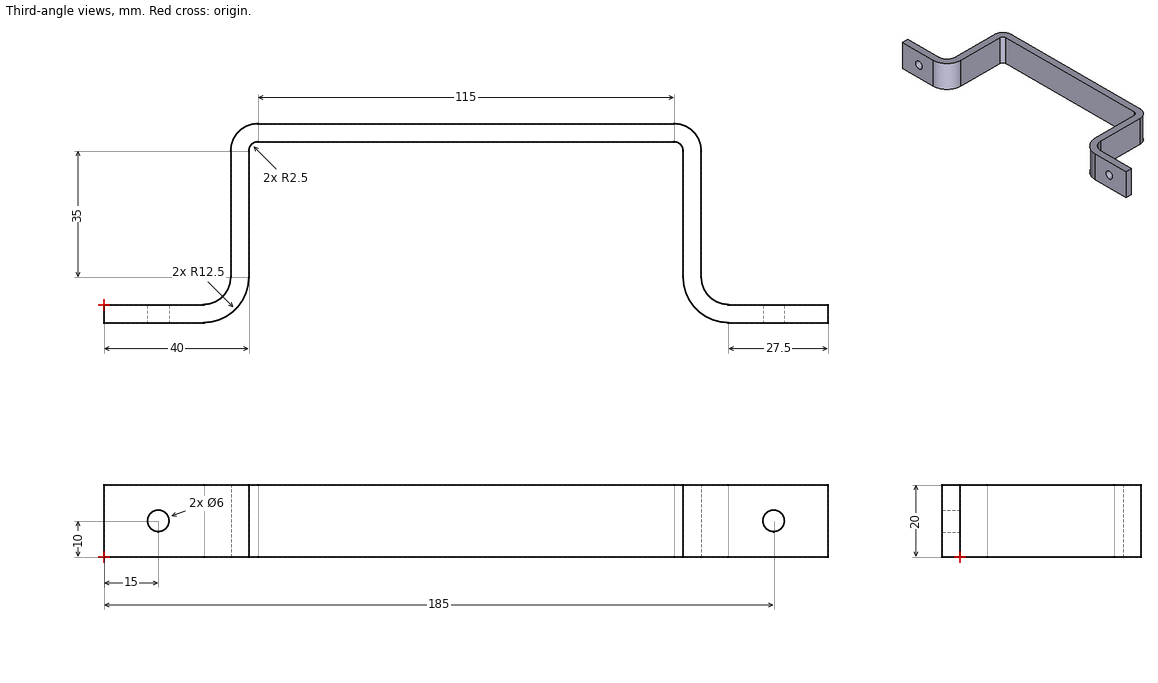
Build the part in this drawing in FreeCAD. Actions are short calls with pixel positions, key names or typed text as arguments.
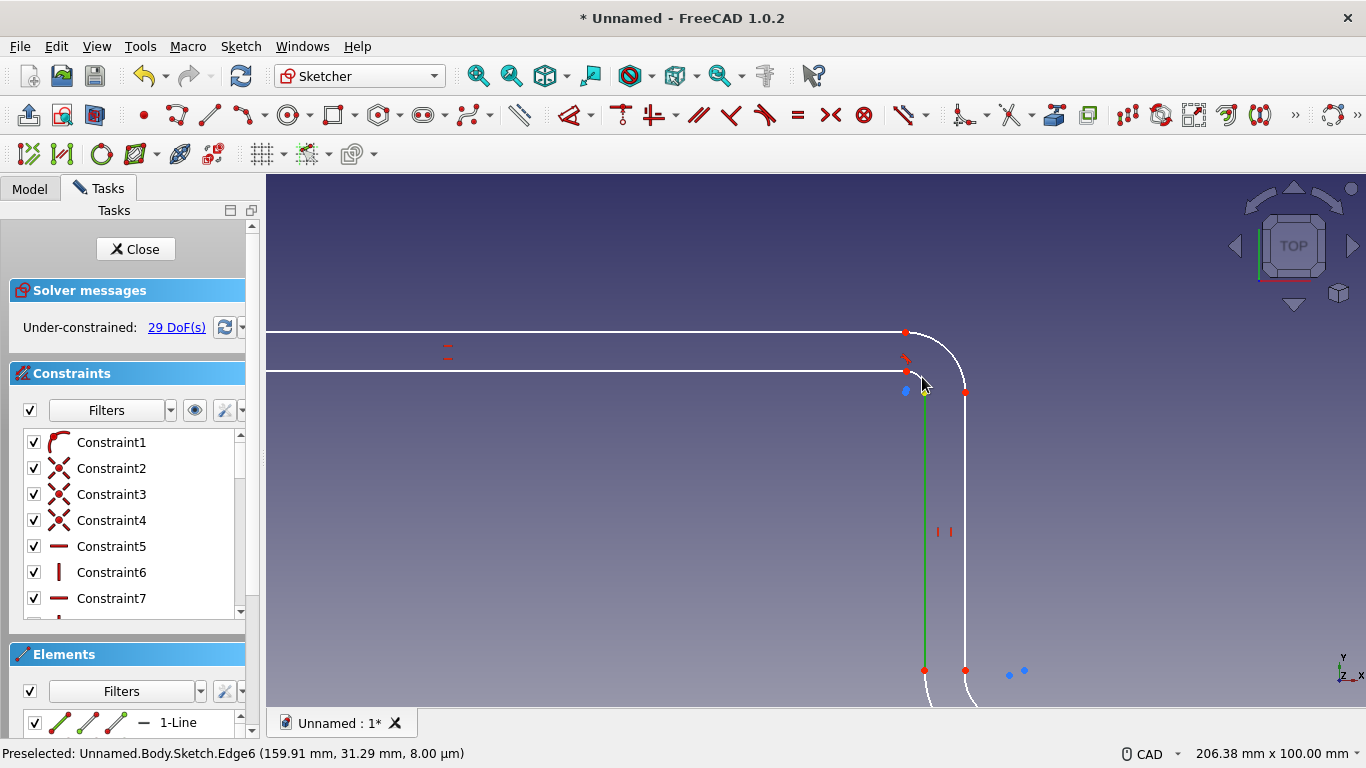
click(920, 378)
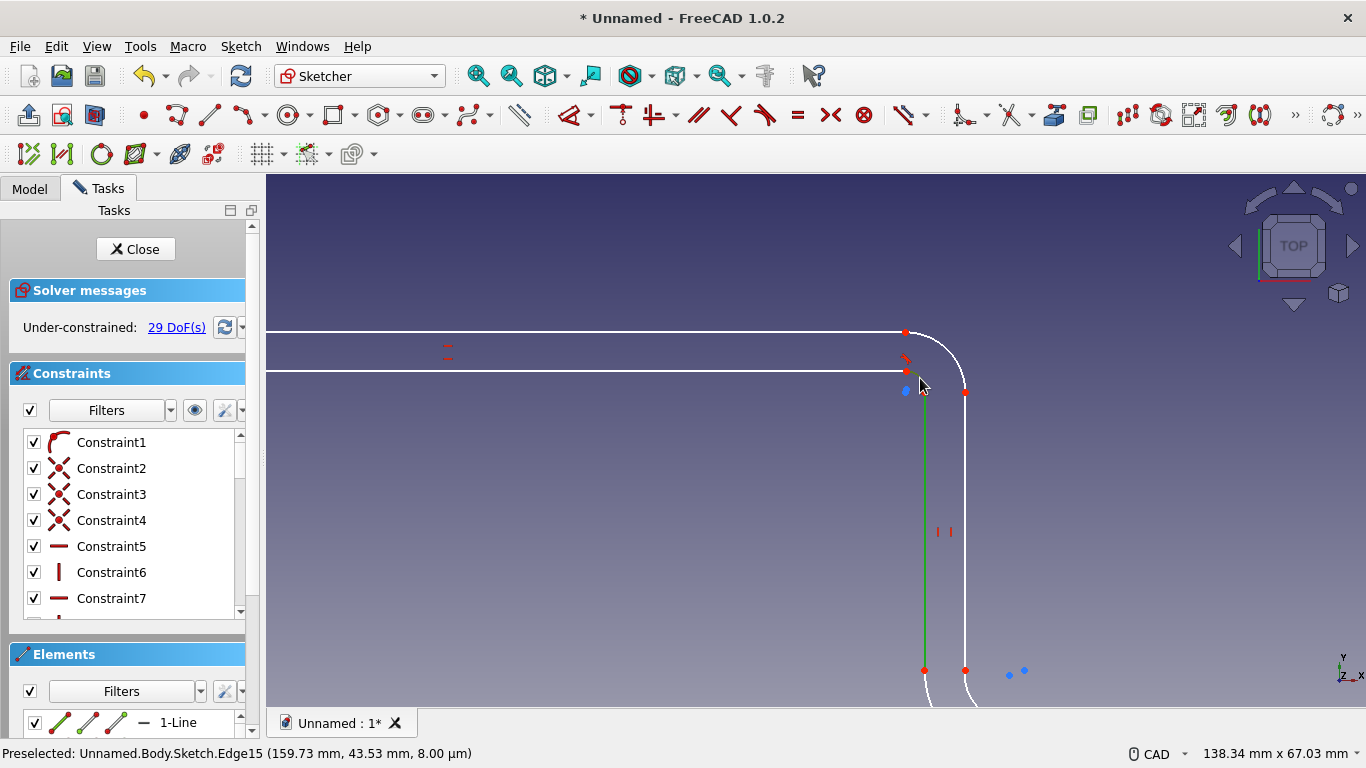
click(765, 116)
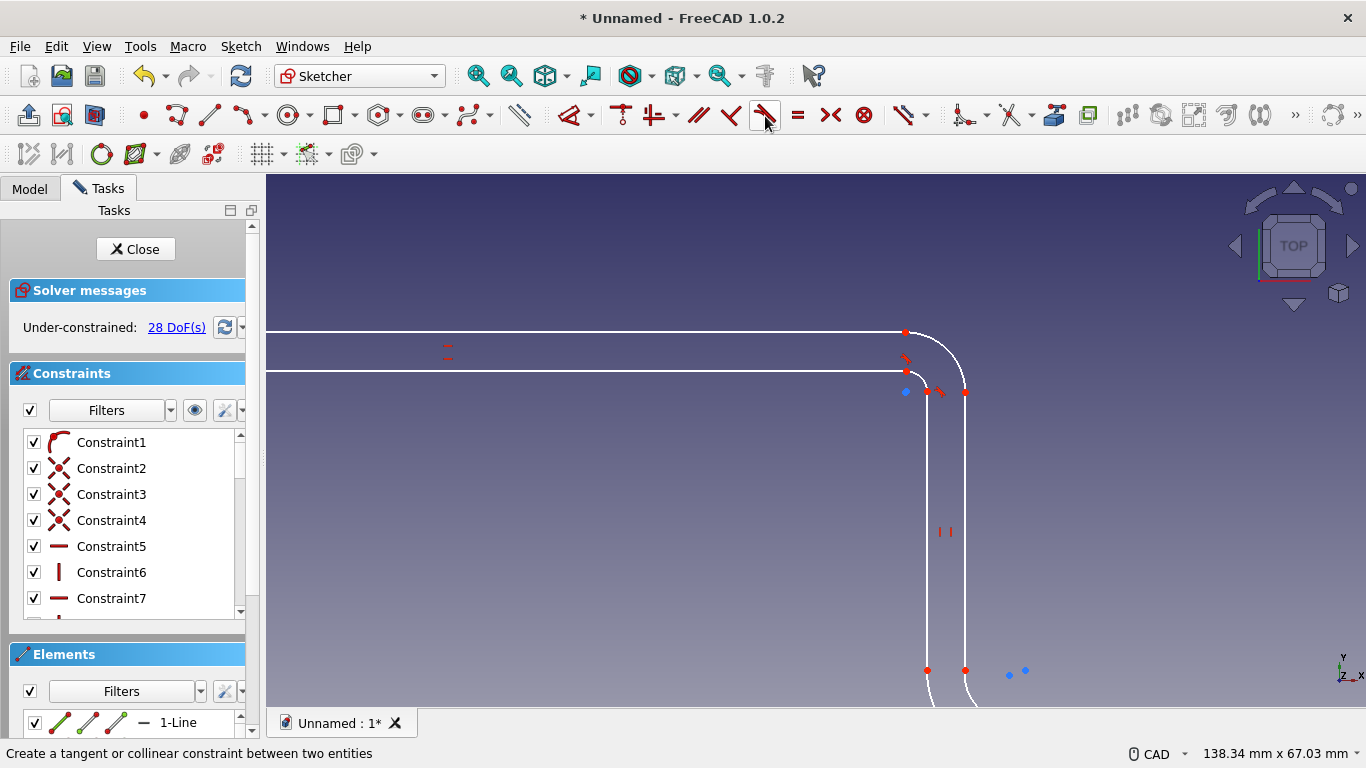
click(927, 476)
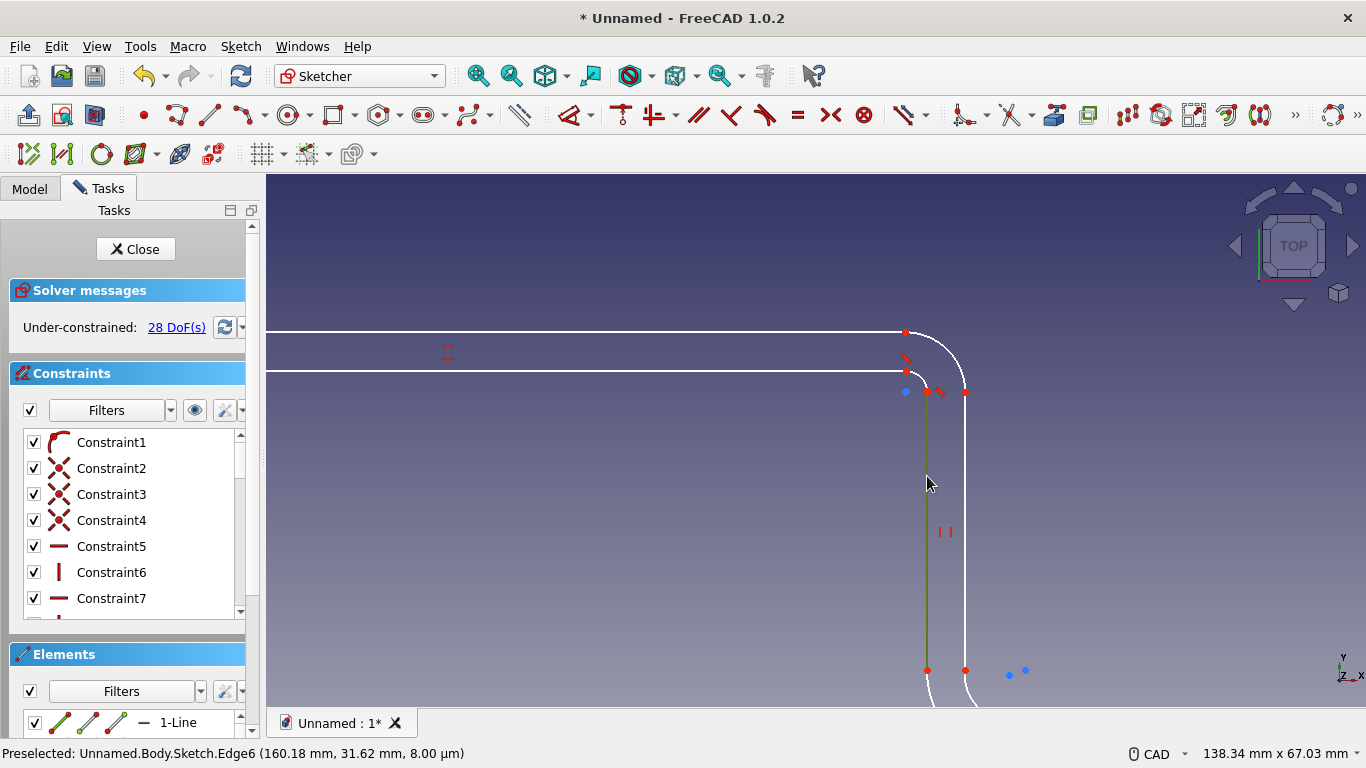
scroll(922, 377, down, 5)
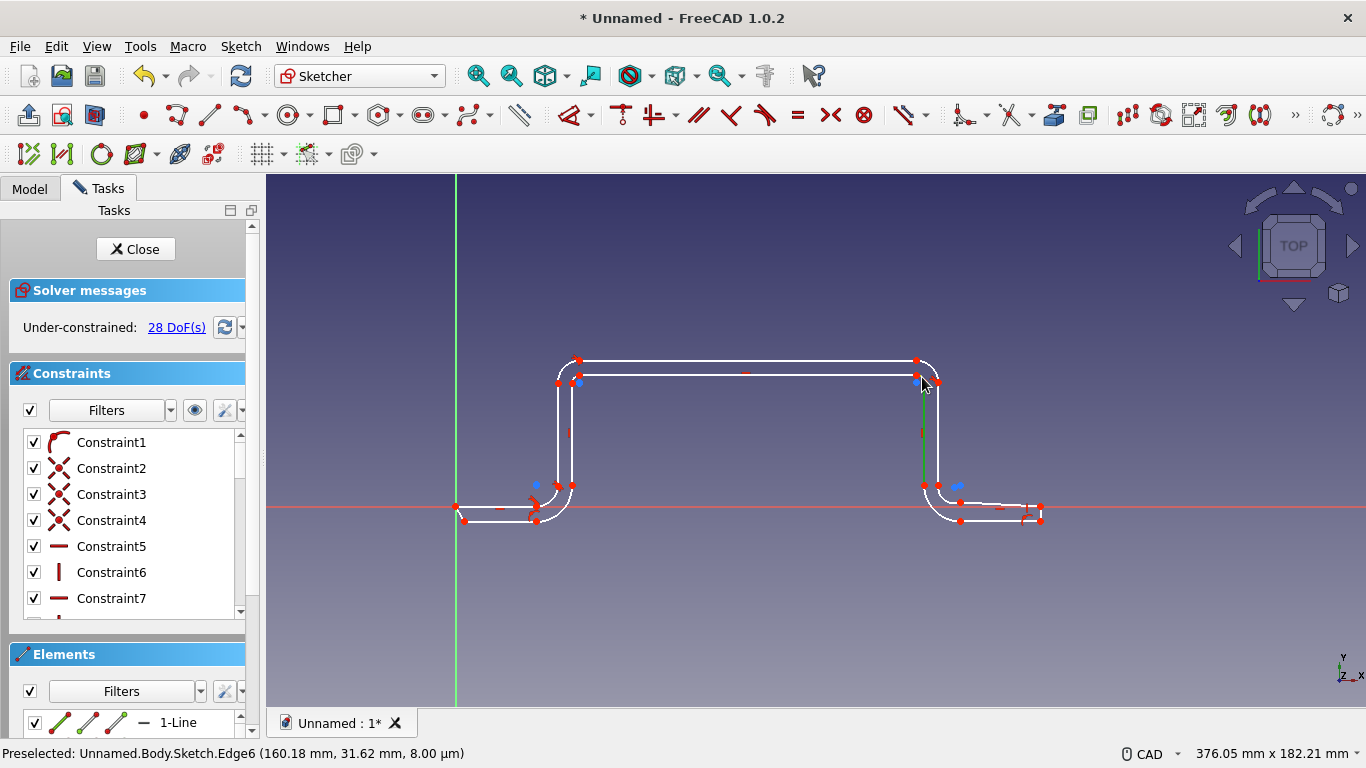
scroll(928, 502, up, 6)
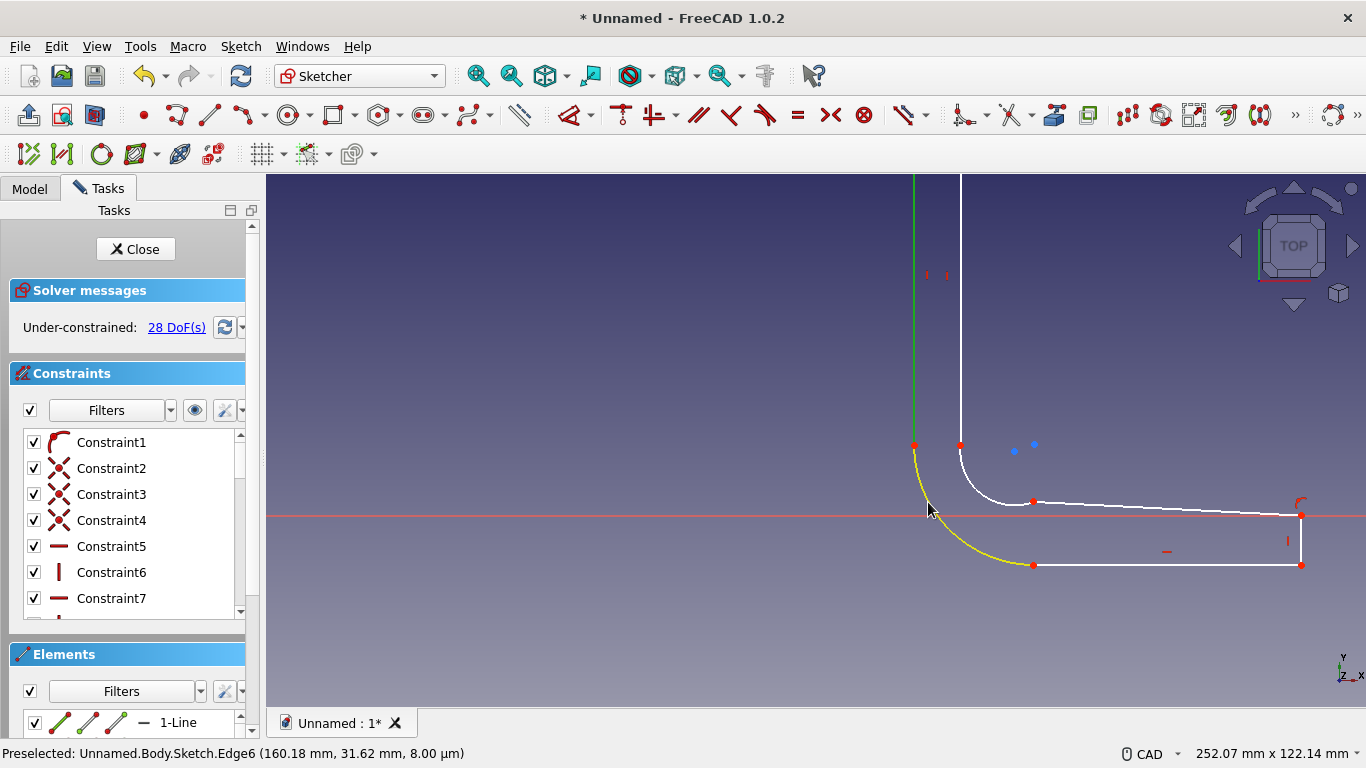
click(927, 499)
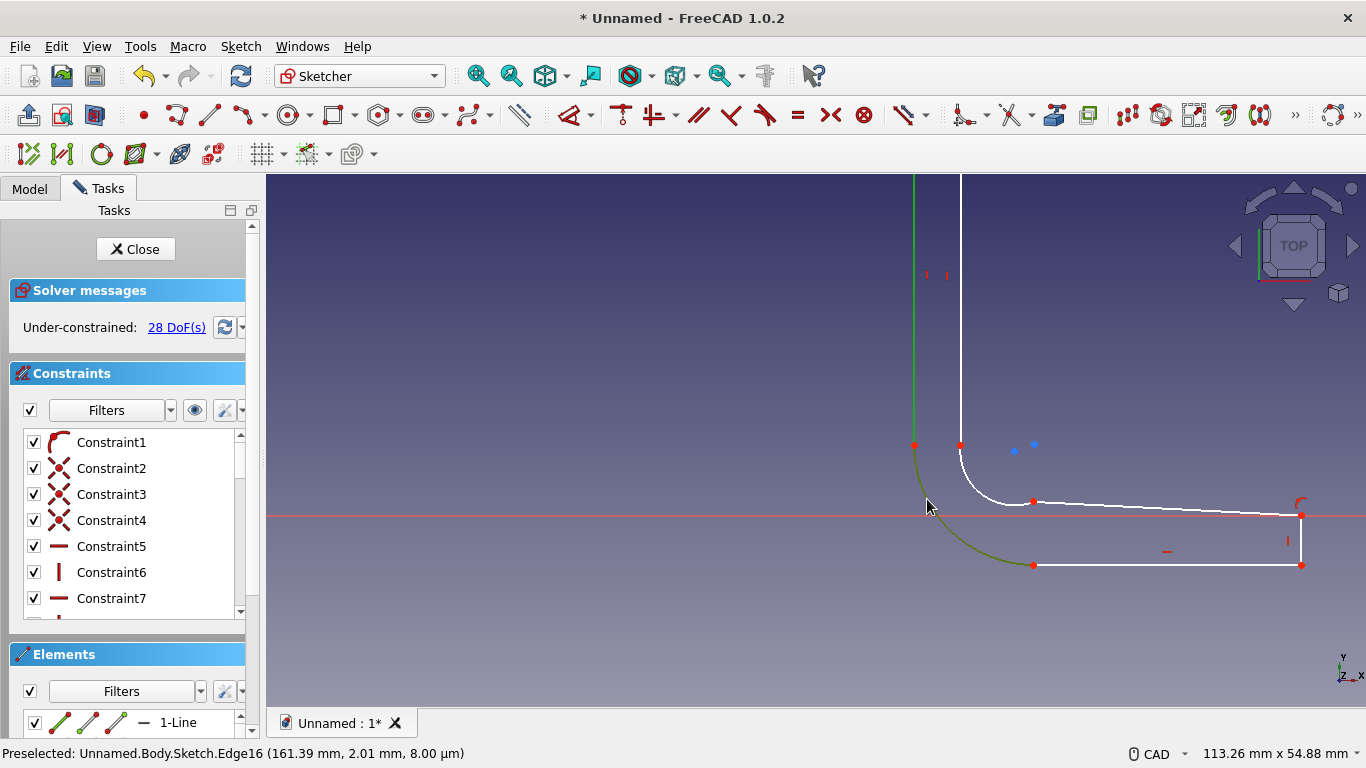
click(765, 116)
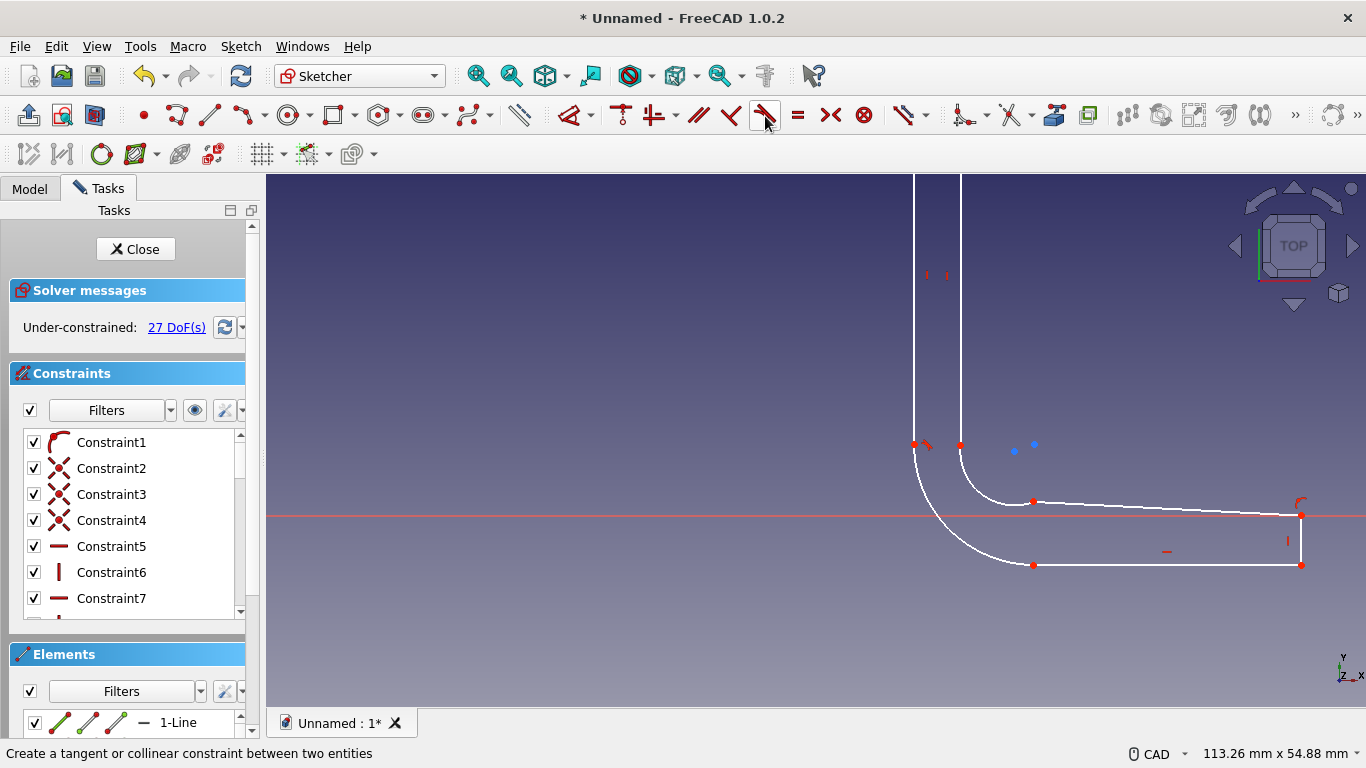
click(1114, 565)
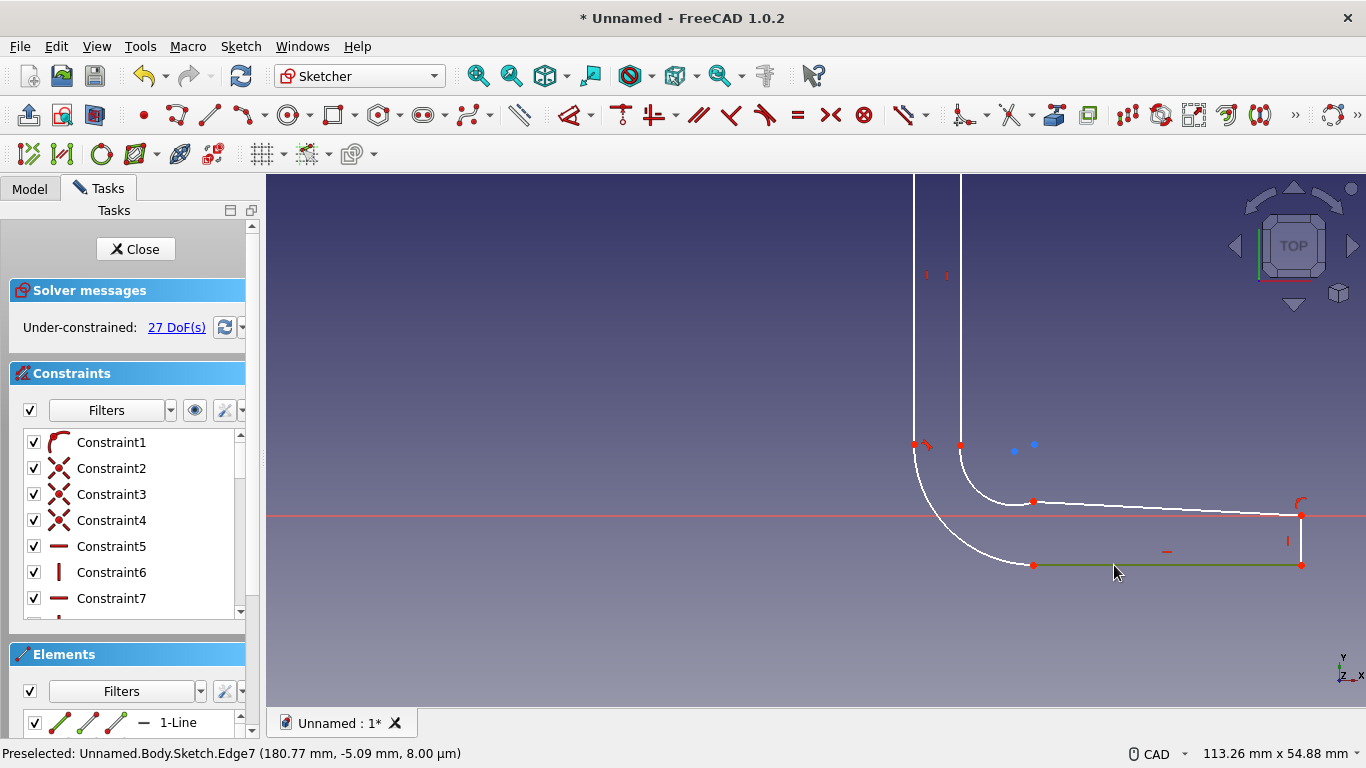
click(927, 499)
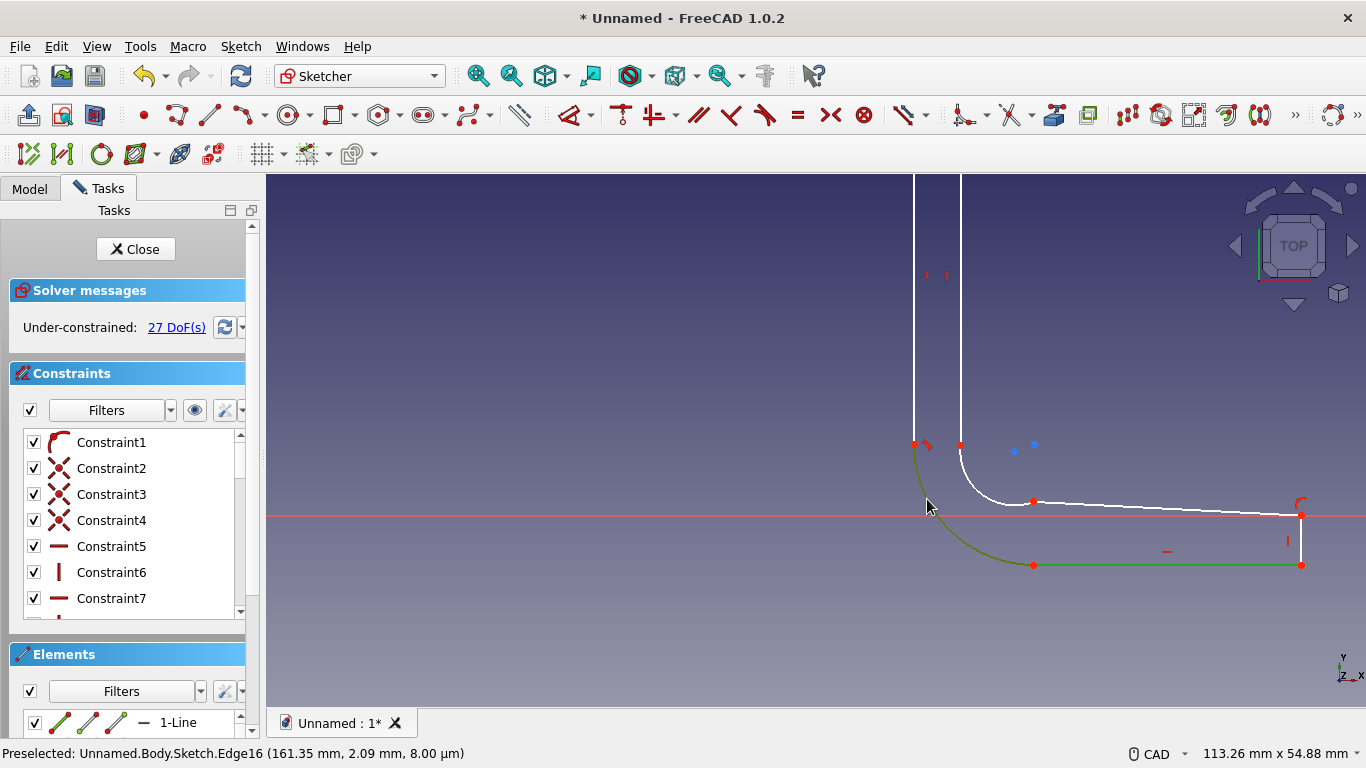
key(t)